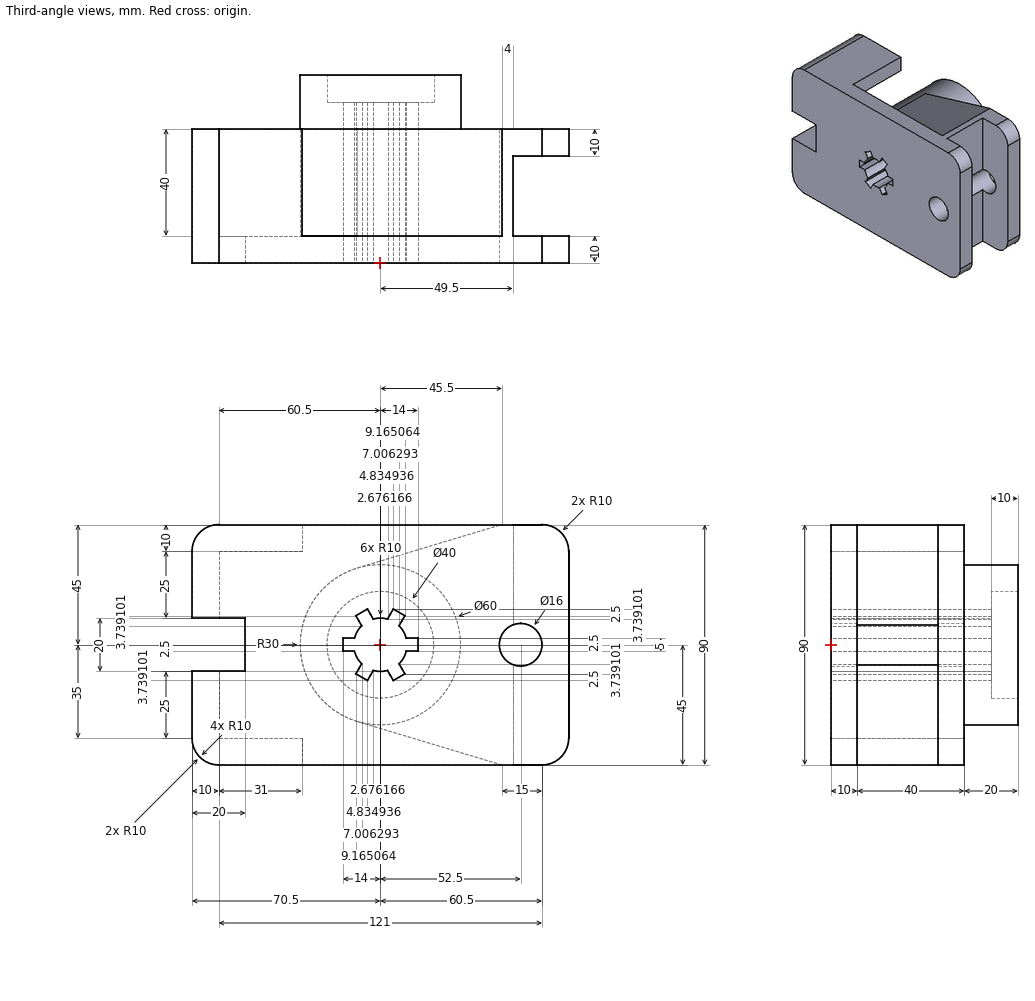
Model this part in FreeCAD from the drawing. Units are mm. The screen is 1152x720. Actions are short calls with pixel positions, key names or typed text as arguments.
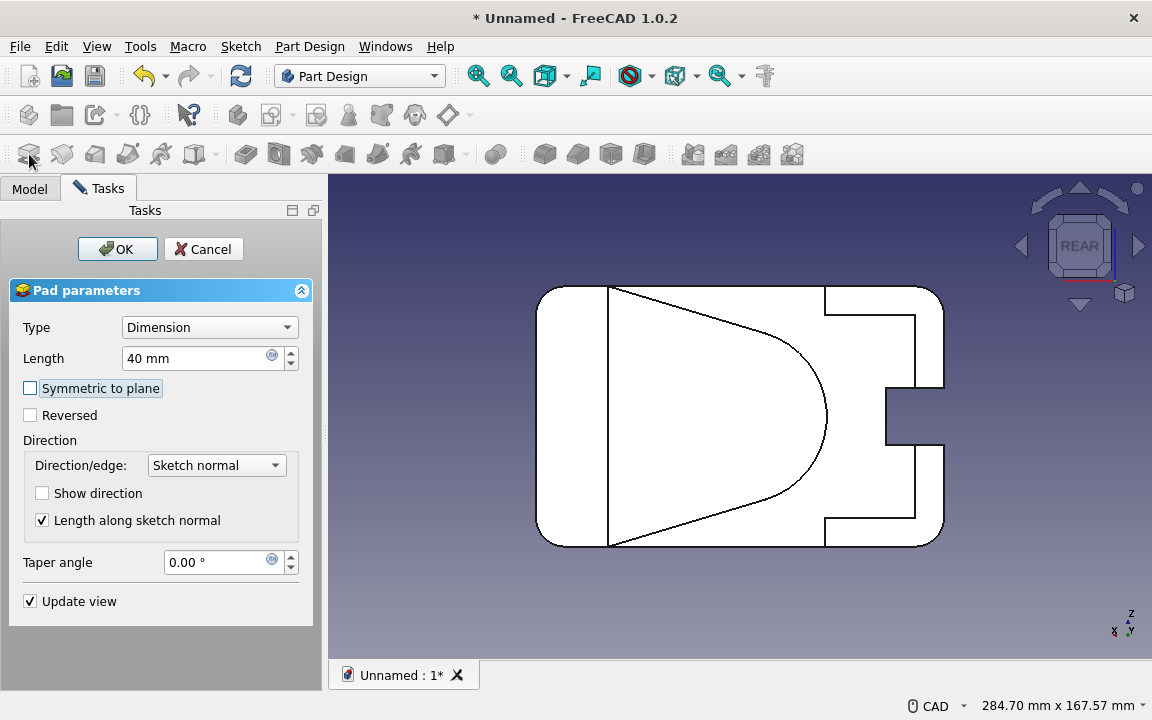
click(118, 249)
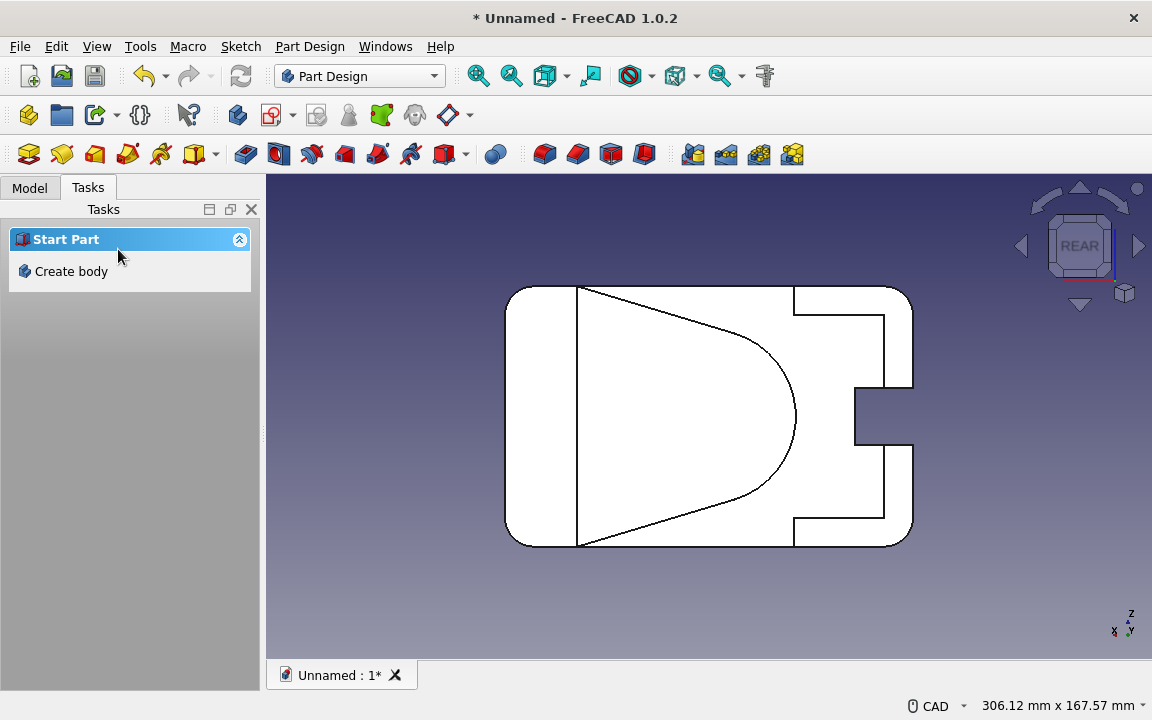
click(30, 188)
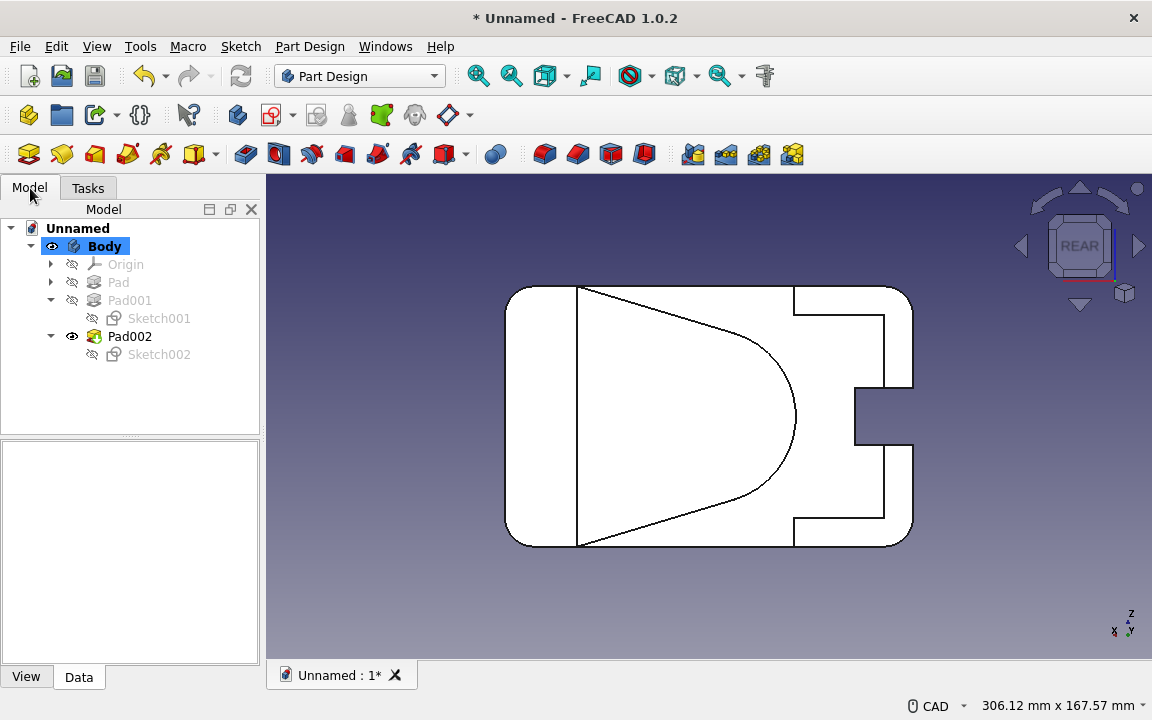
click(51, 264)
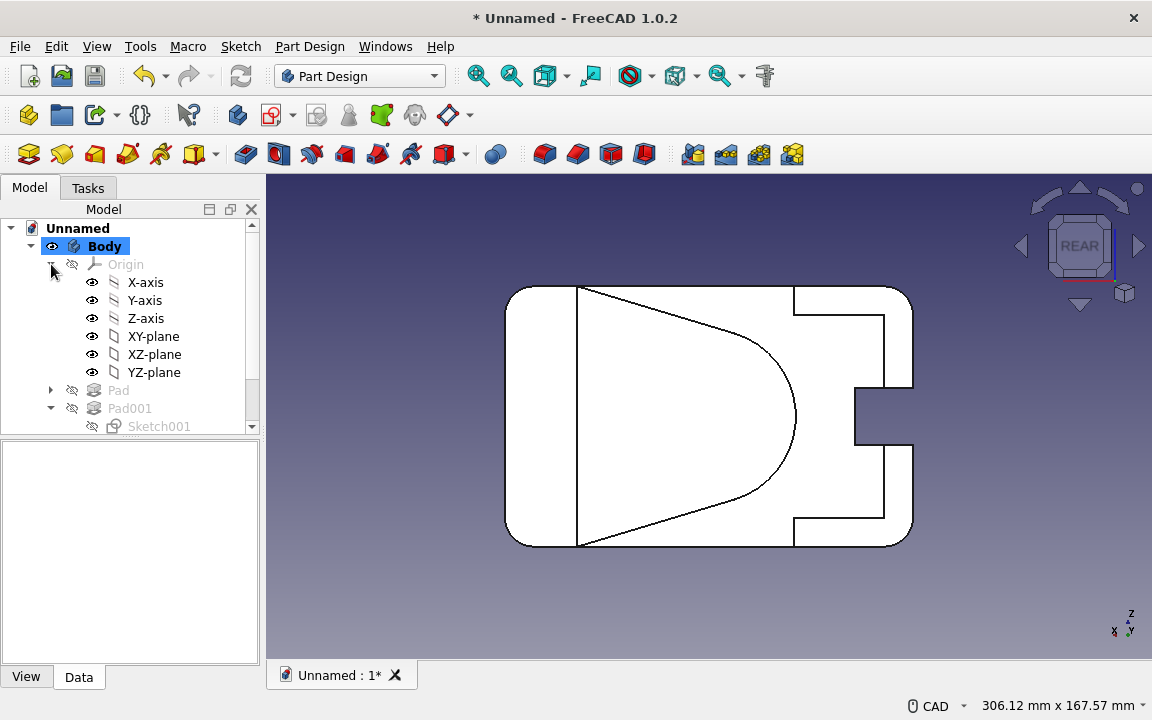
click(137, 354)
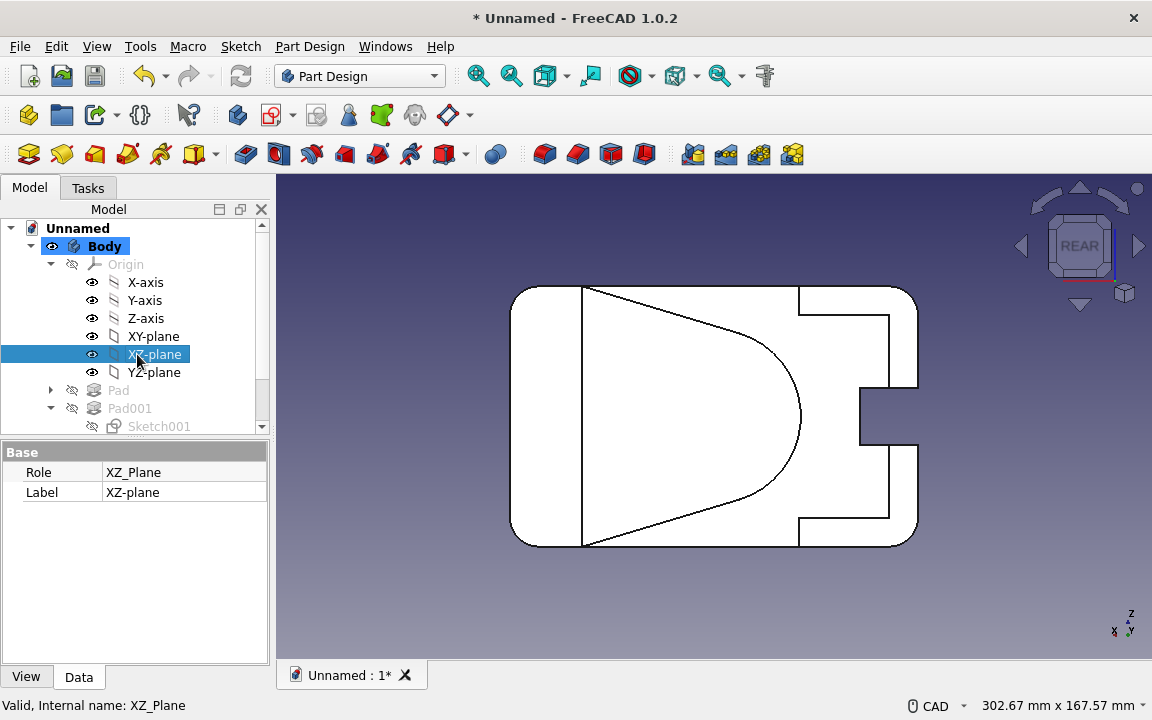
click(448, 116)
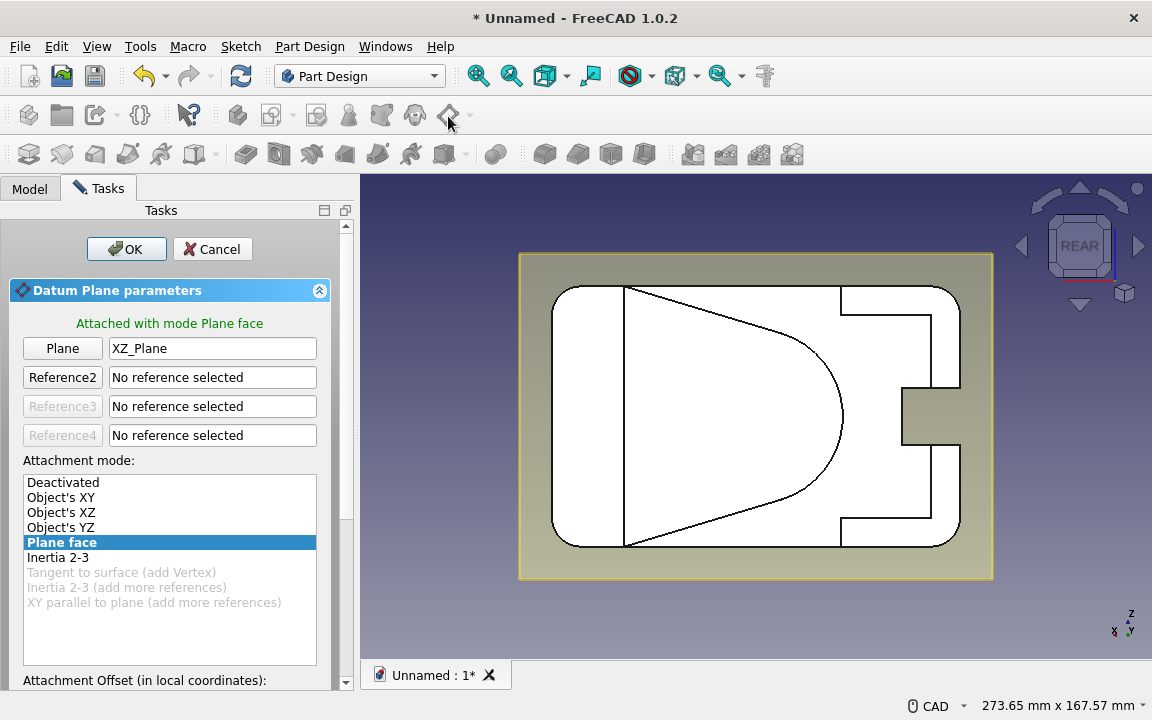
scroll(346, 455, down, 3)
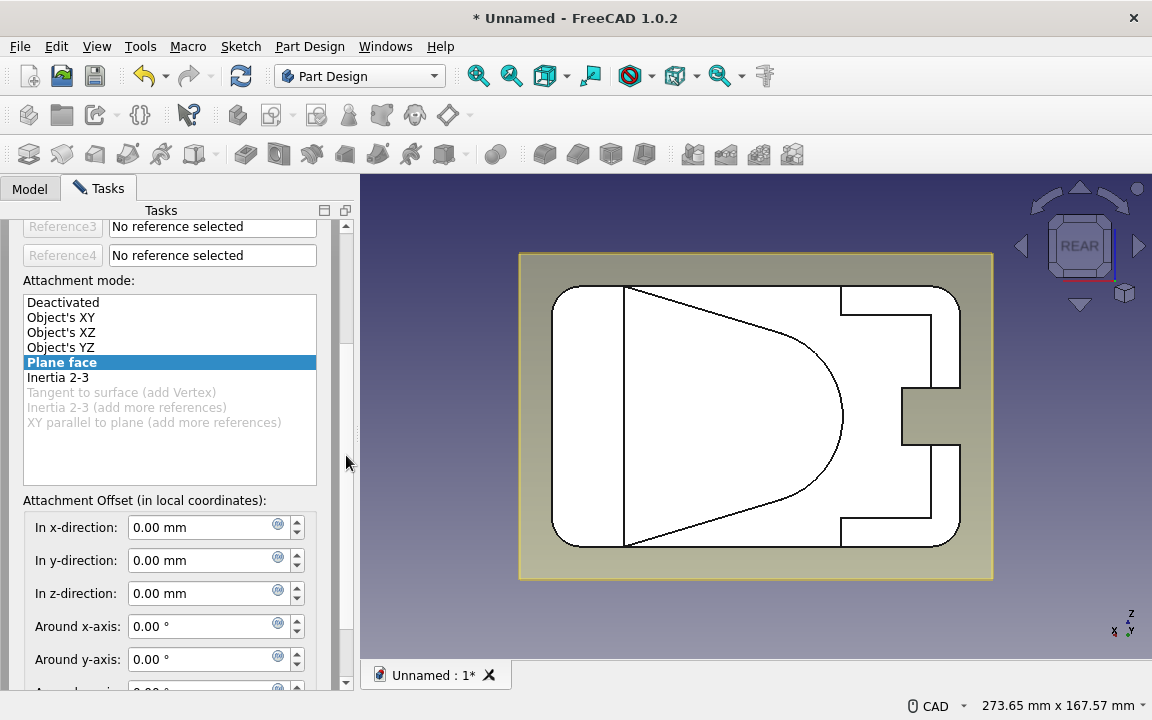
triple_click(210, 594)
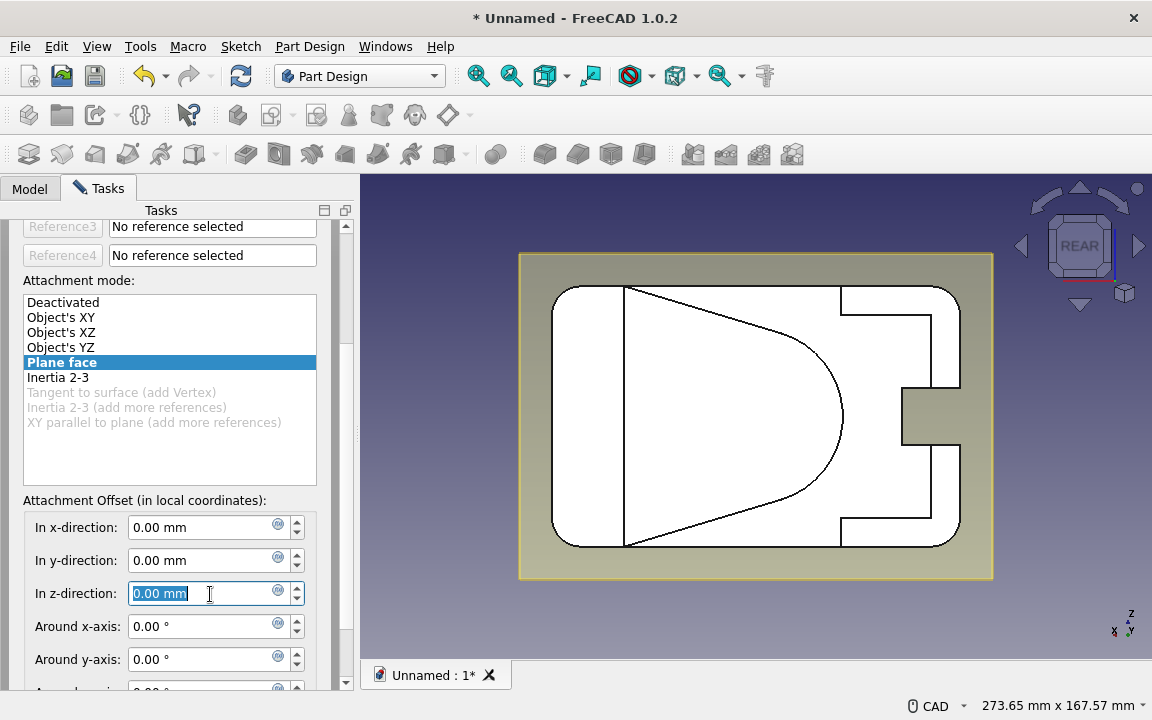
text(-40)
key(Tab)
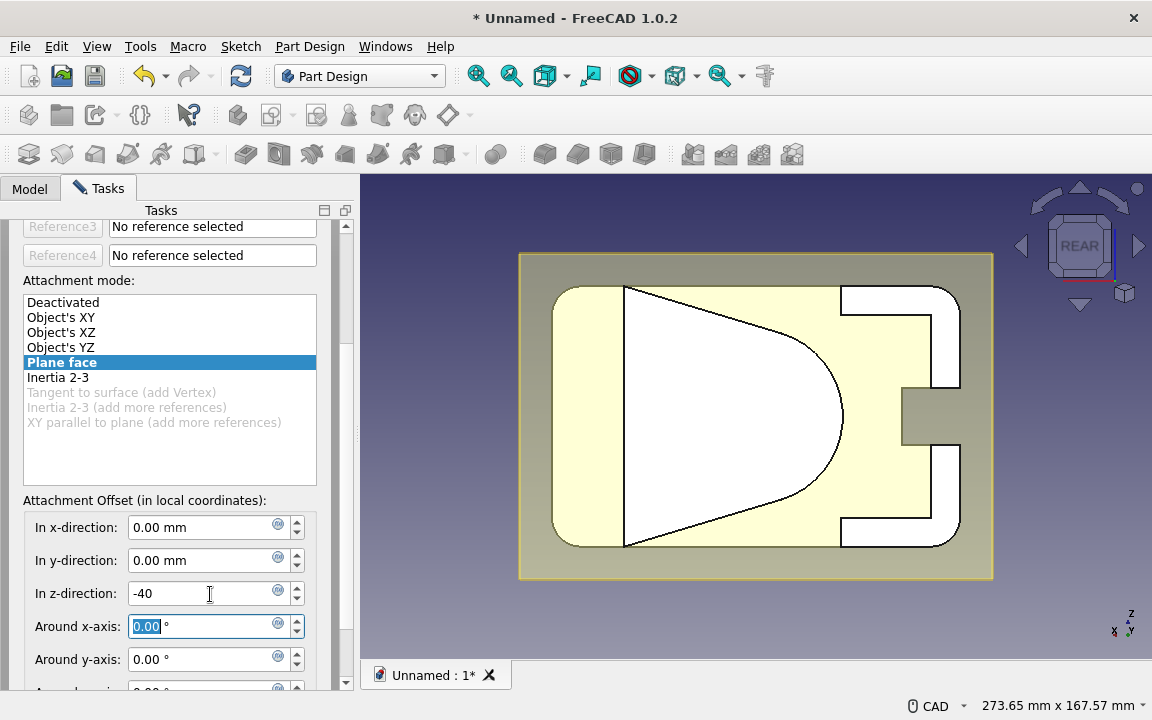
scroll(346, 455, up, 4)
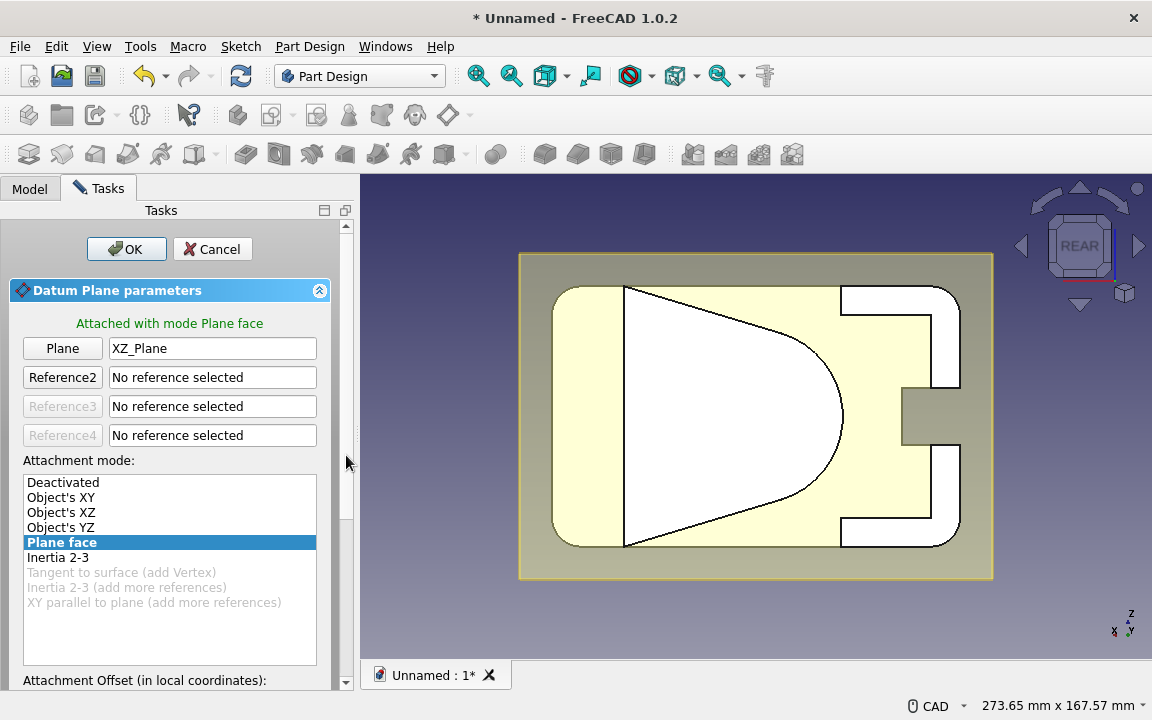
click(127, 249)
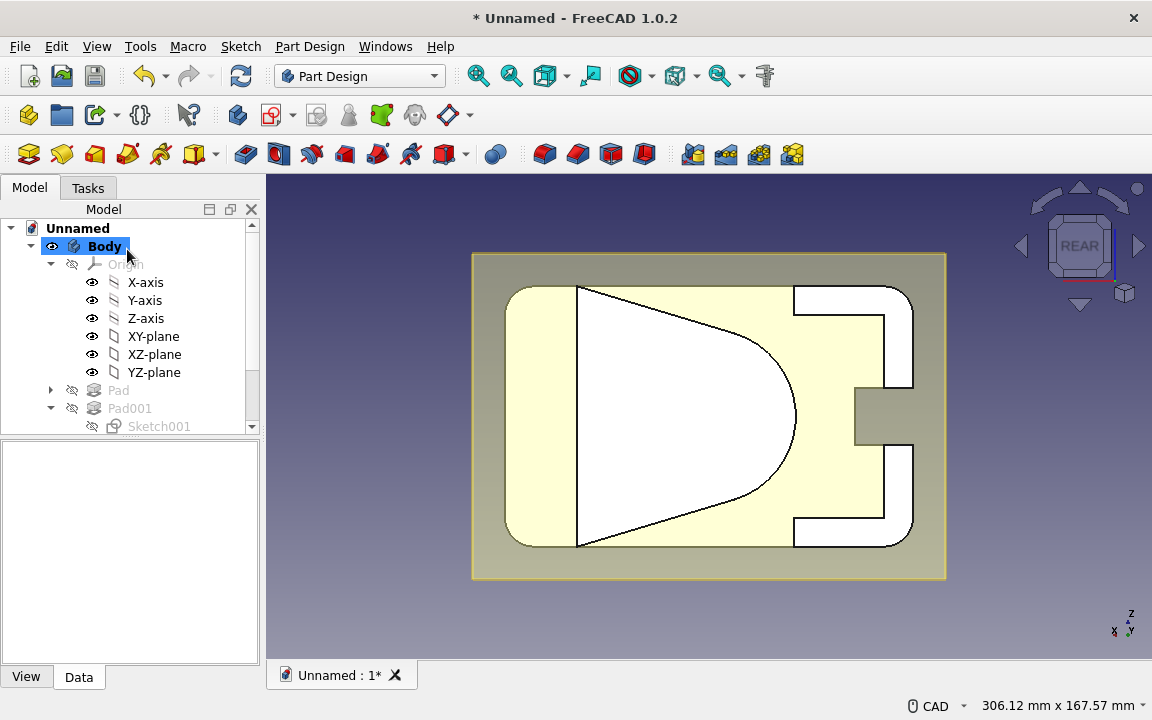
scroll(101, 332, down, 3)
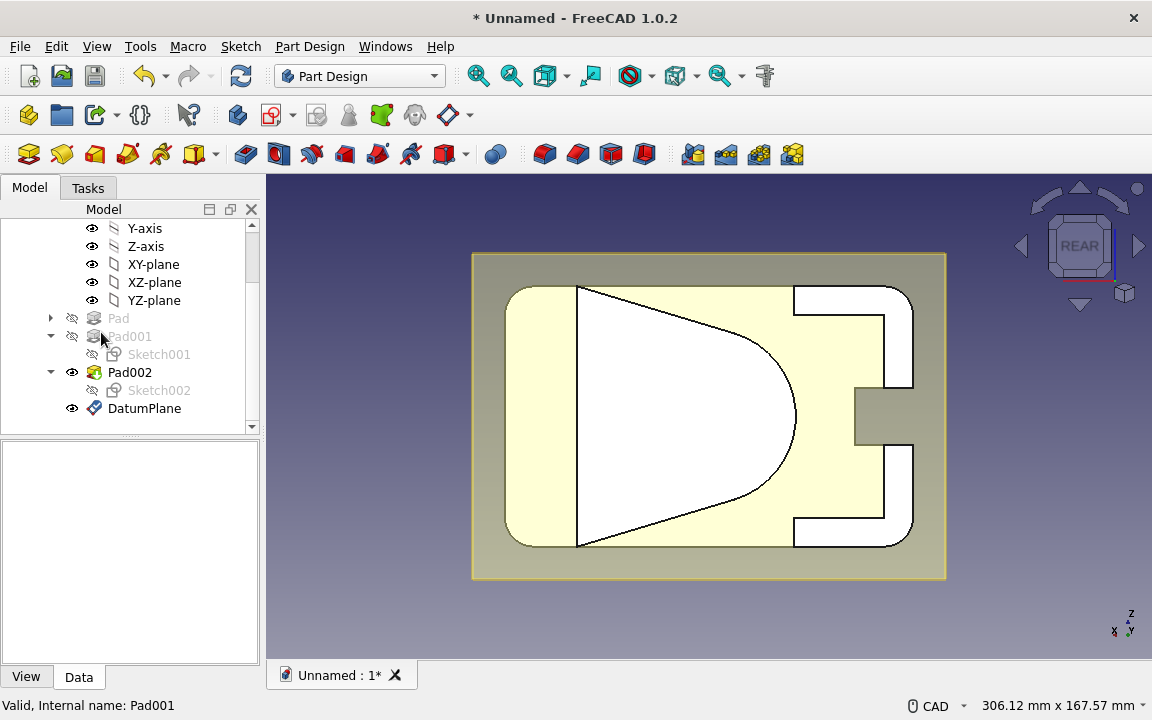
click(117, 408)